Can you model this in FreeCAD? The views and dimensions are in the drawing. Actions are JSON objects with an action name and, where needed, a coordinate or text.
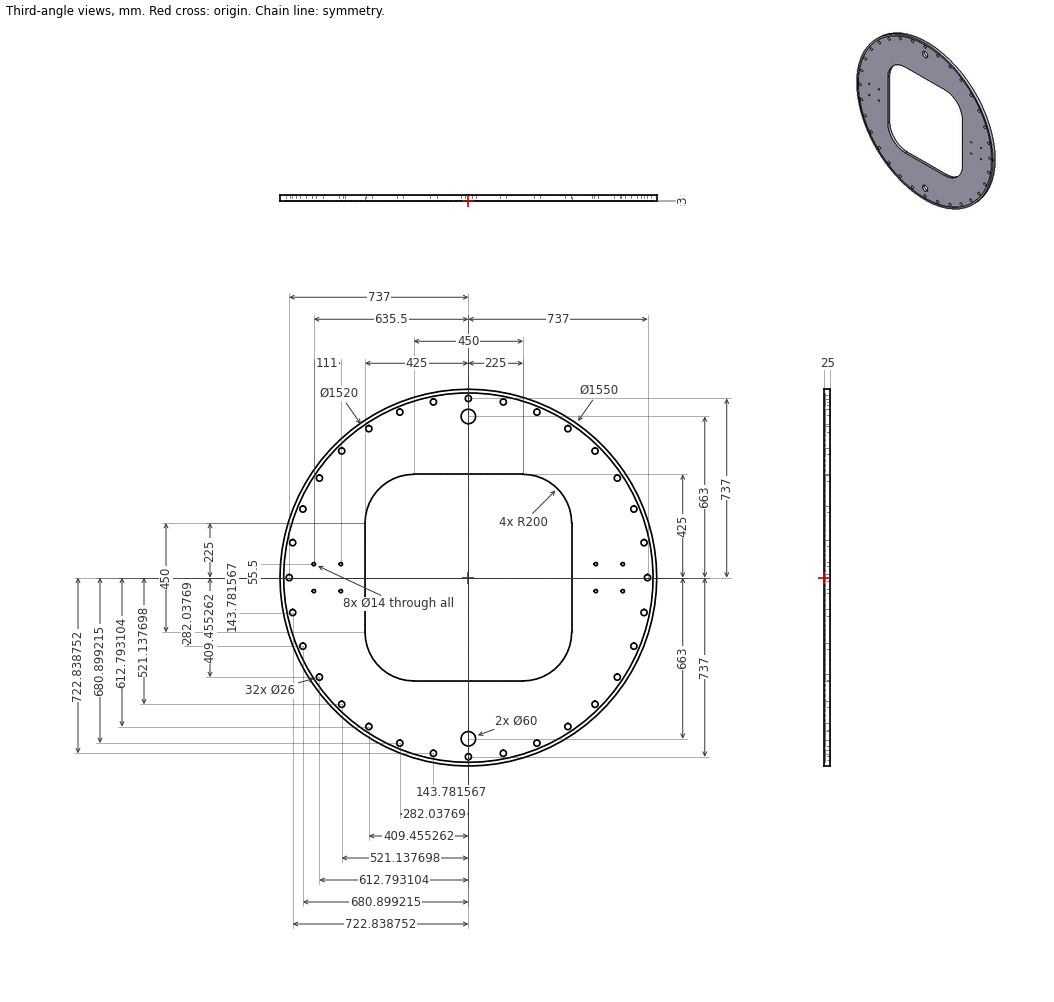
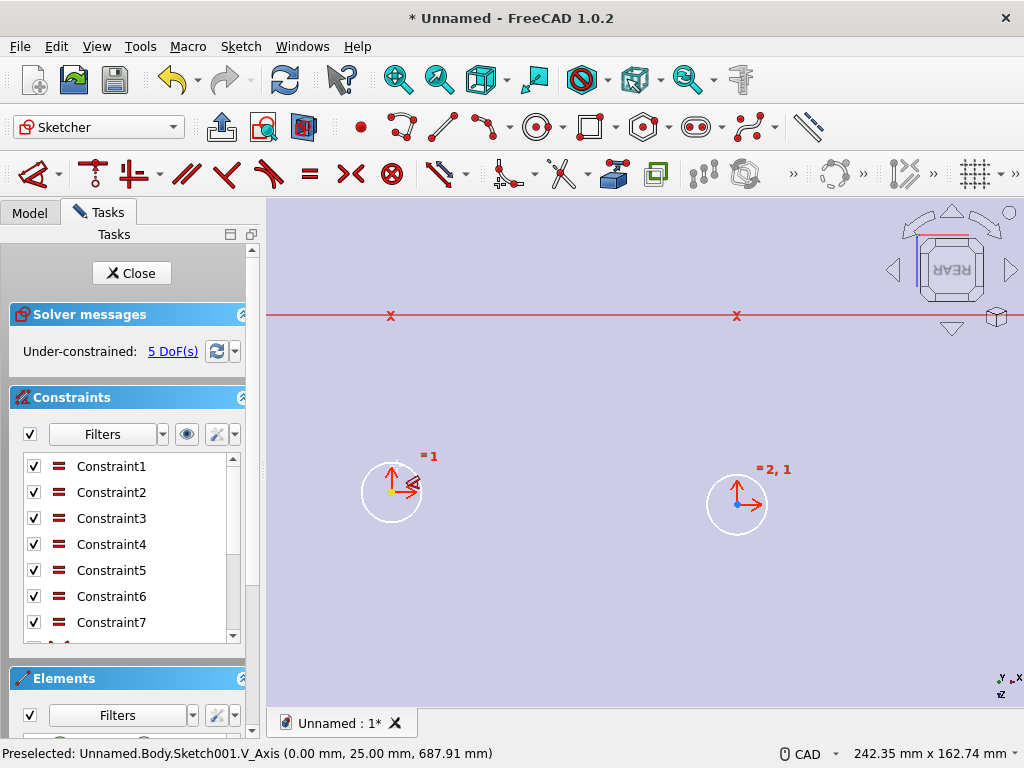
{"action": "left_click", "coordinate": [392, 463]}
{"action": "left_click", "coordinate": [392, 431]}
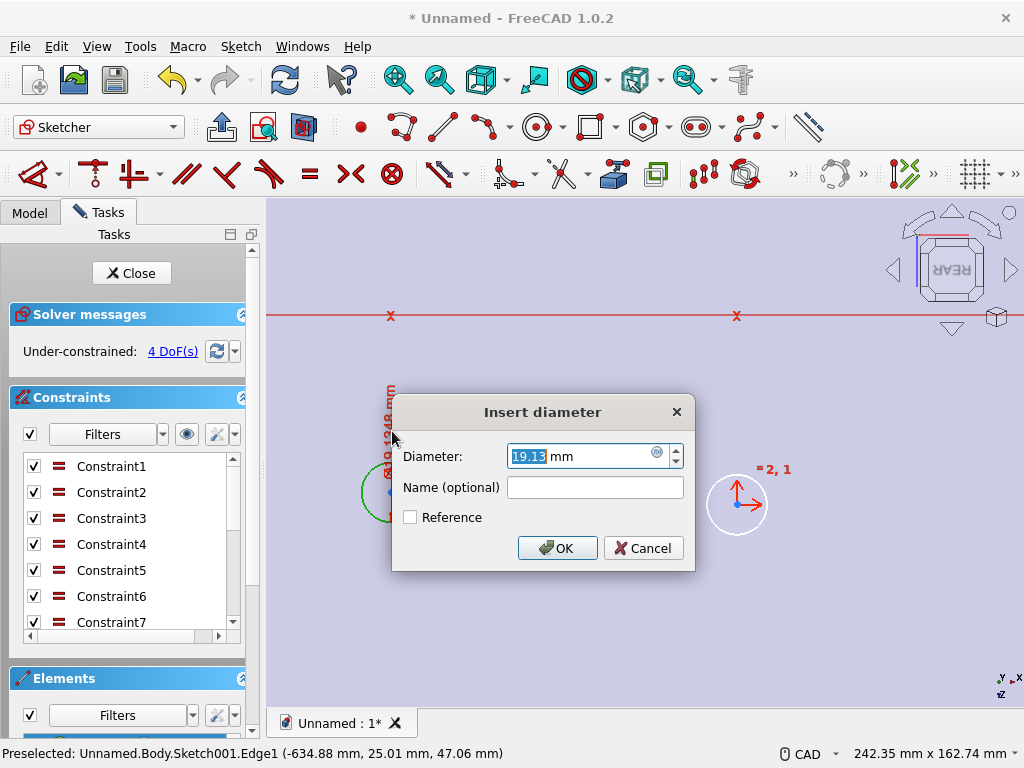
{"action": "type", "text": "14"}
{"action": "key", "text": "Return"}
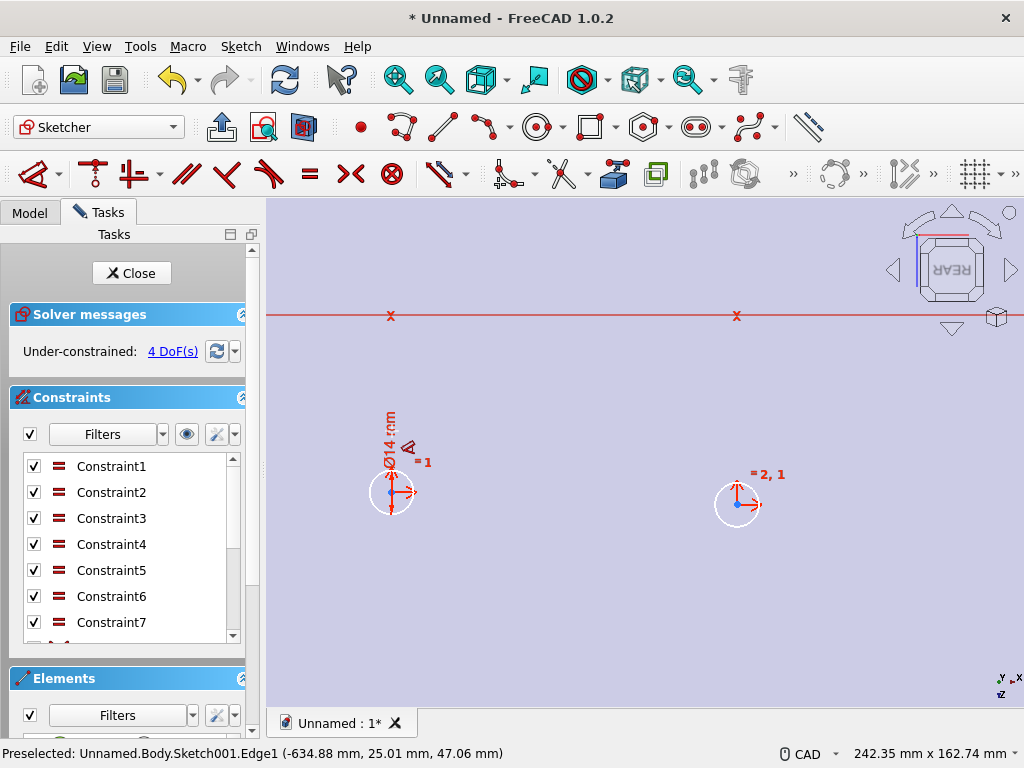
{"action": "scroll", "coordinate": [397, 466], "scroll_direction": "down", "scroll_amount": 12}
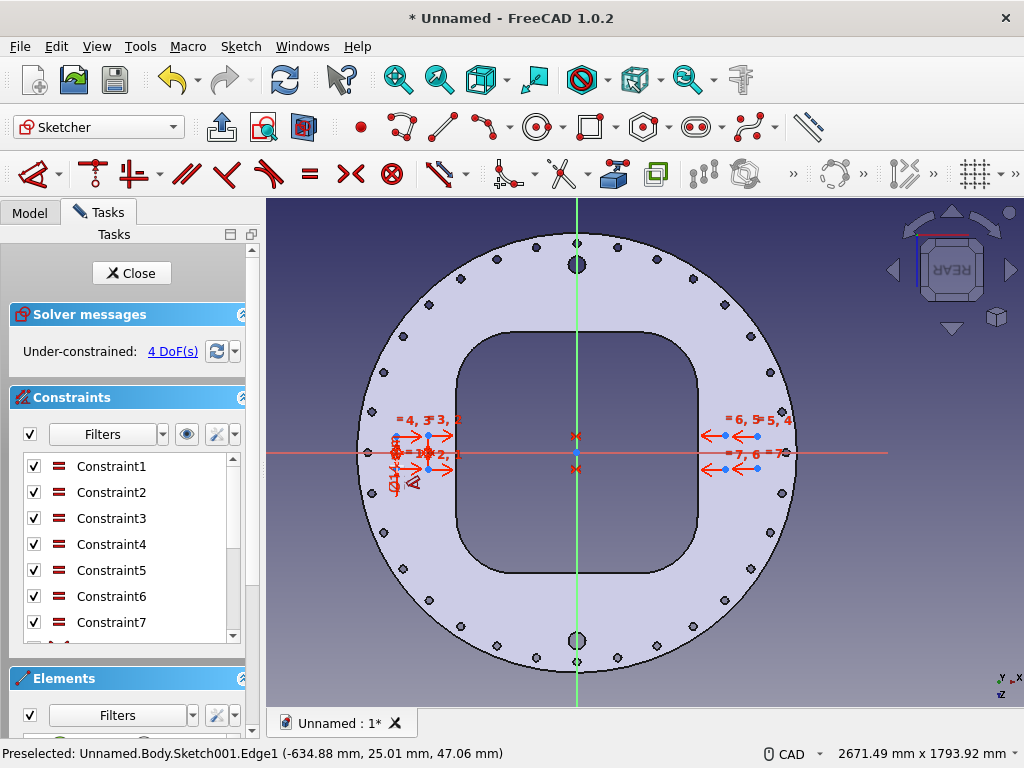
{"action": "scroll", "coordinate": [397, 469], "scroll_direction": "up", "scroll_amount": 5}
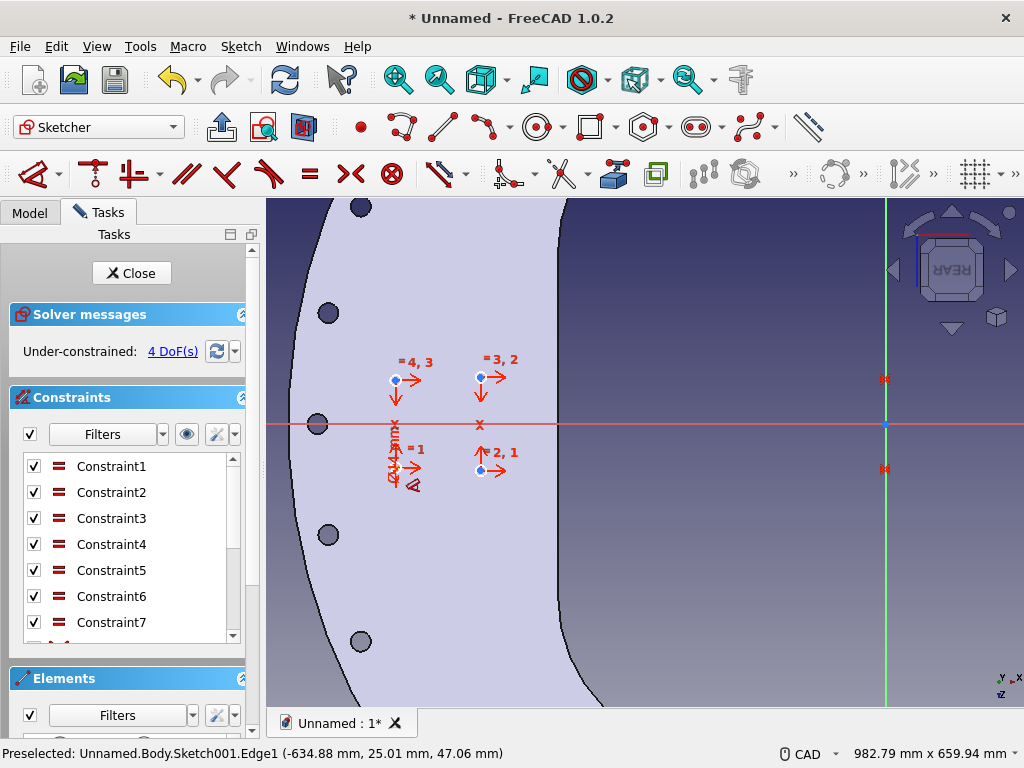
{"action": "left_click", "coordinate": [396, 468]}
{"action": "left_click", "coordinate": [314, 446]}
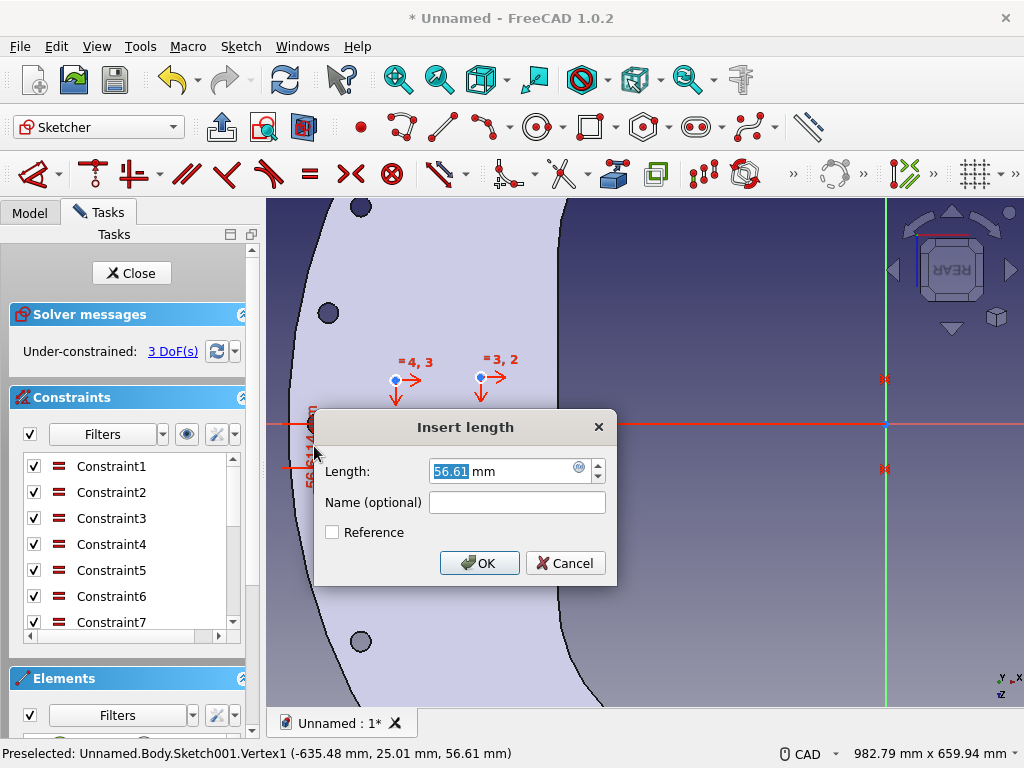
{"action": "type", "text": "55.5"}
{"action": "key", "text": "Return"}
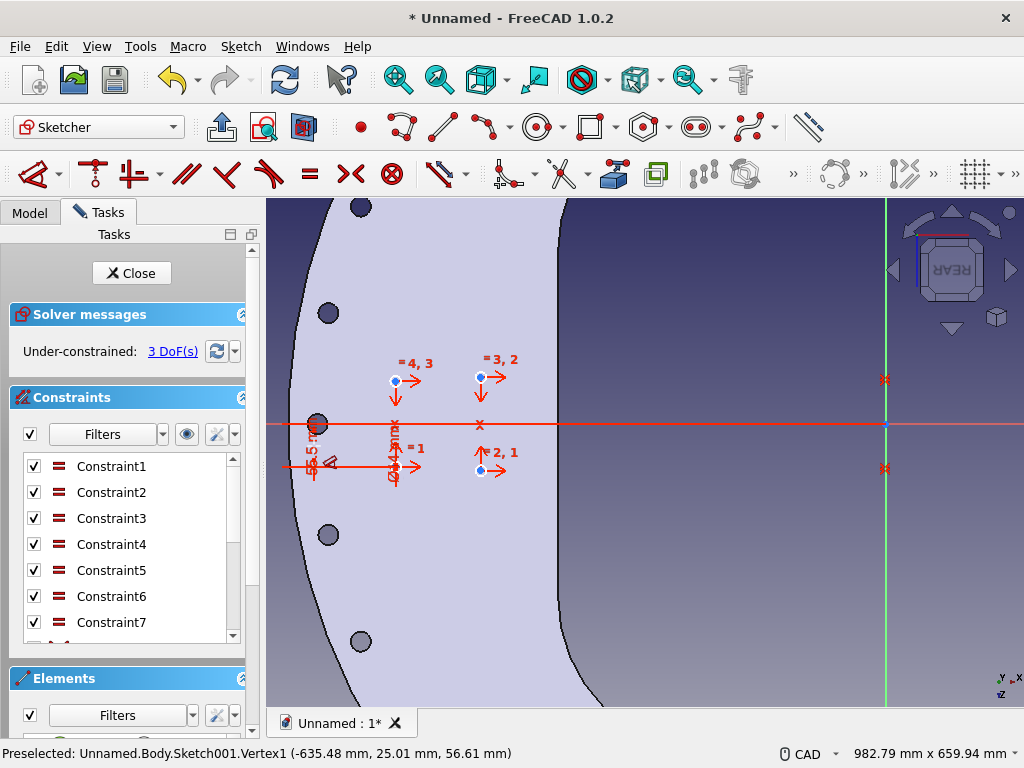
{"action": "left_click", "coordinate": [481, 471]}
{"action": "left_click", "coordinate": [447, 447]}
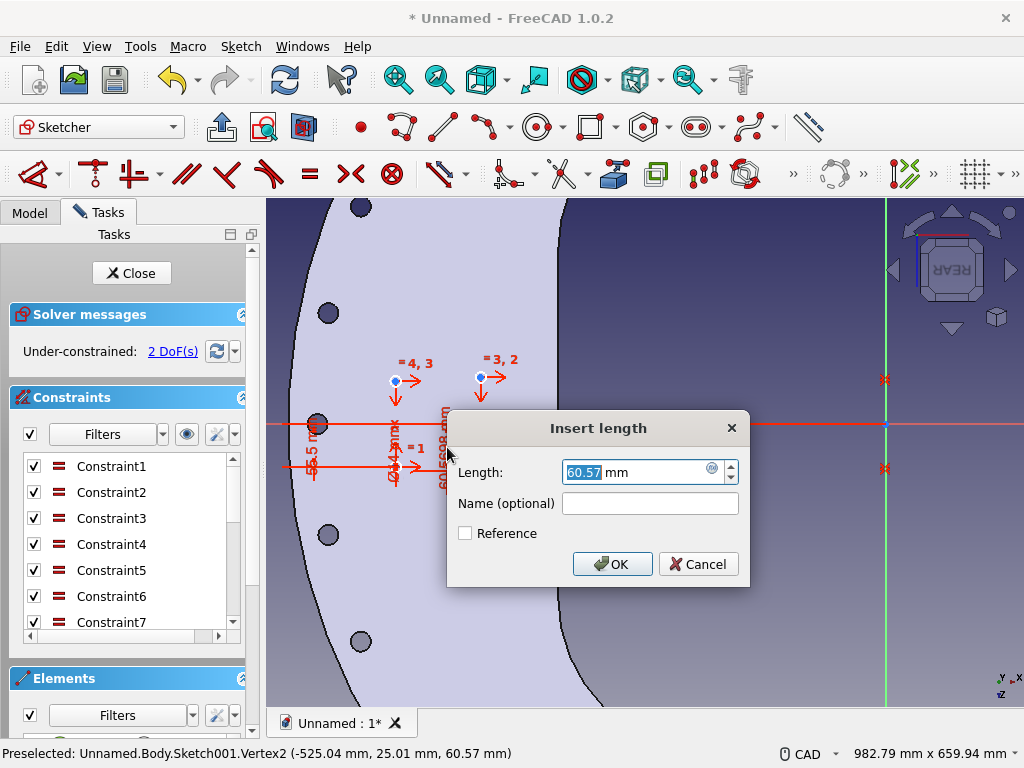
{"action": "type", "text": "55.5"}
{"action": "key", "text": "Return"}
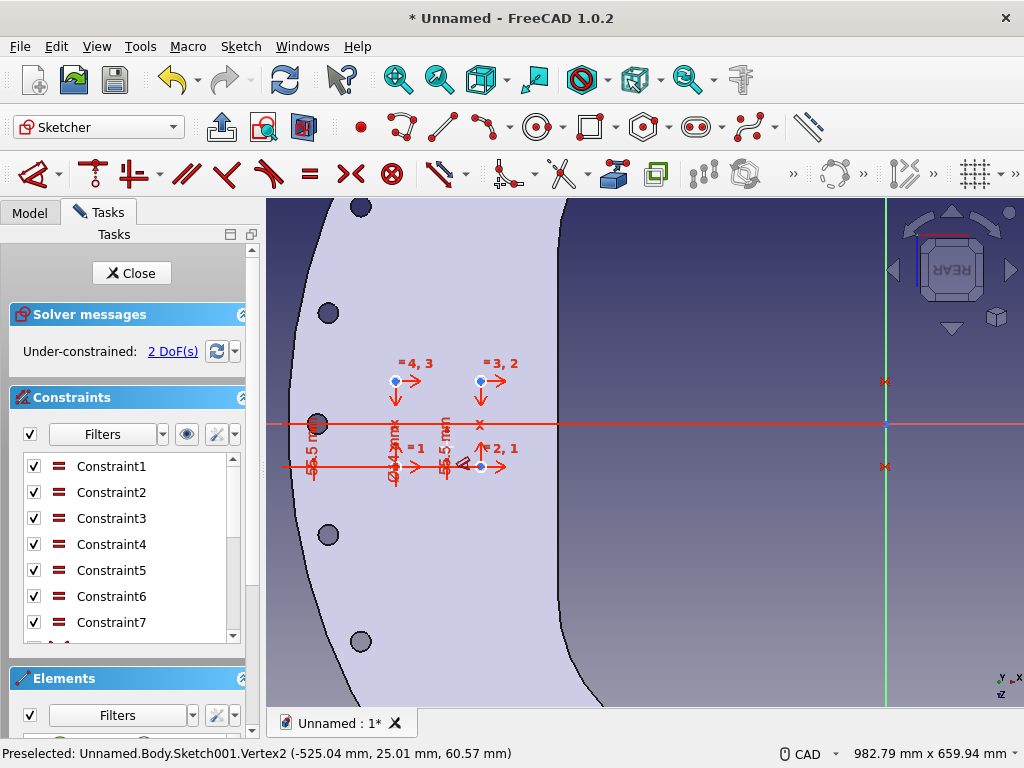
{"action": "left_click", "coordinate": [396, 467]}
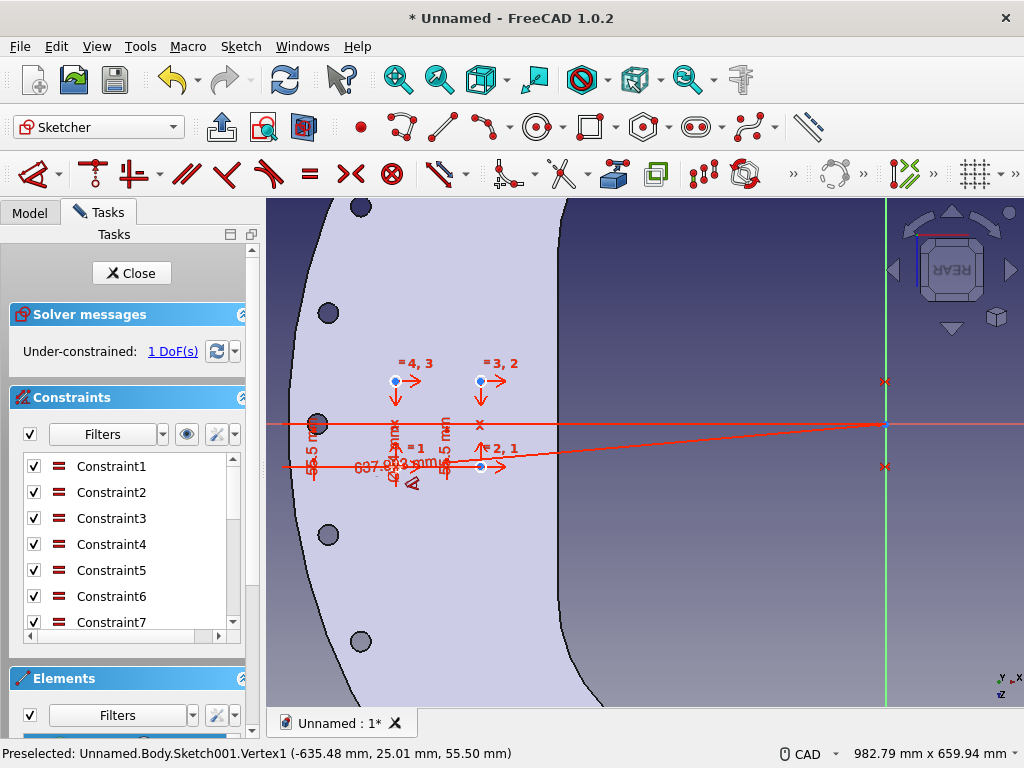
{"action": "left_click", "coordinate": [481, 467]}
{"action": "left_click", "coordinate": [438, 501]}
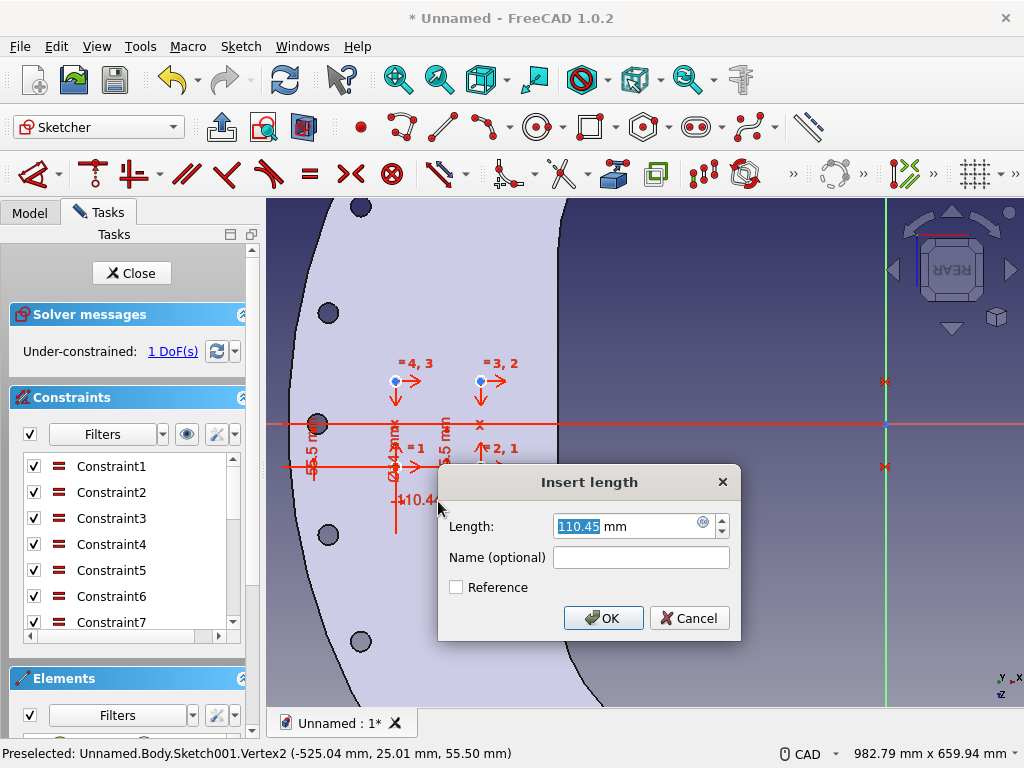
{"action": "type", "text": "111"}
{"action": "key", "text": "Return"}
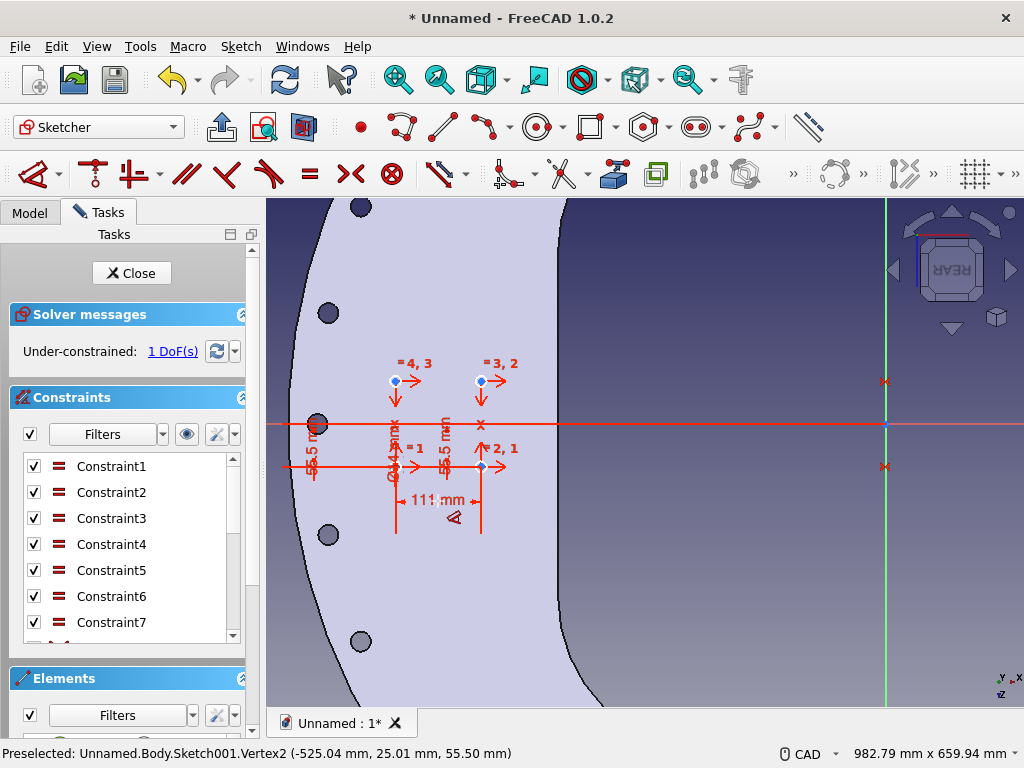
{"action": "left_click", "coordinate": [396, 467]}
{"action": "left_click", "coordinate": [627, 501]}